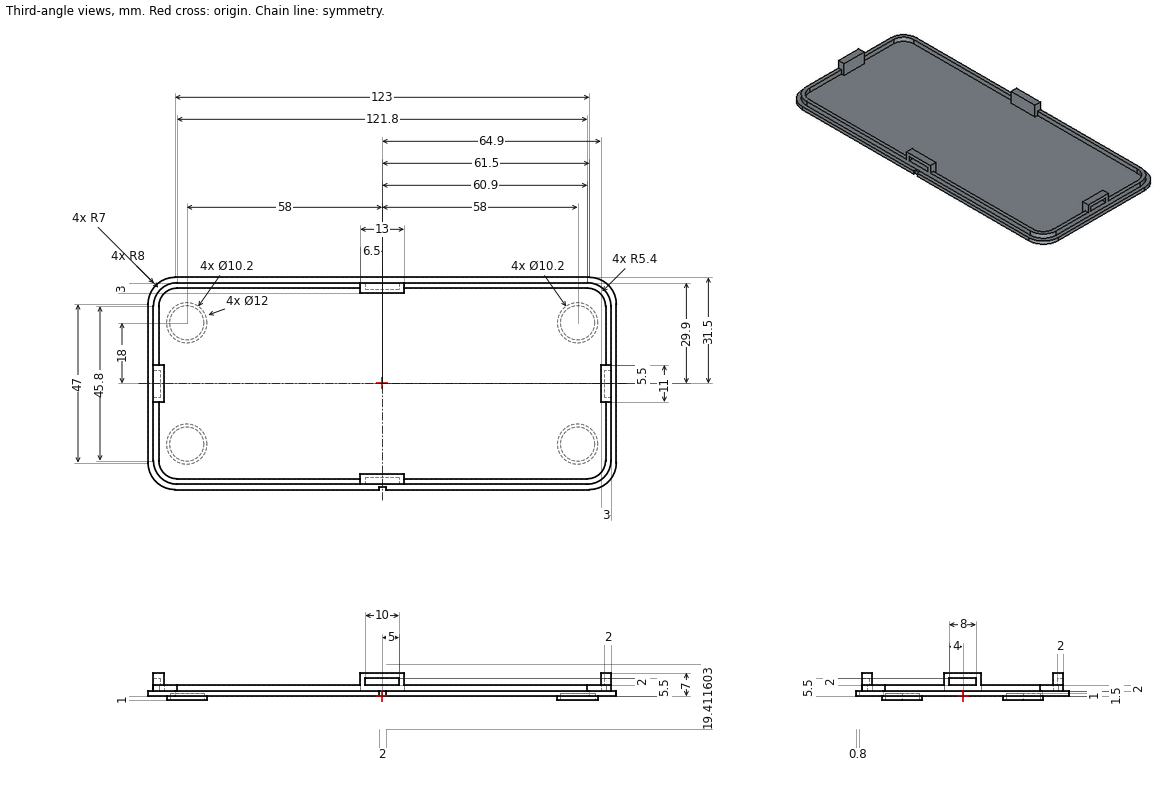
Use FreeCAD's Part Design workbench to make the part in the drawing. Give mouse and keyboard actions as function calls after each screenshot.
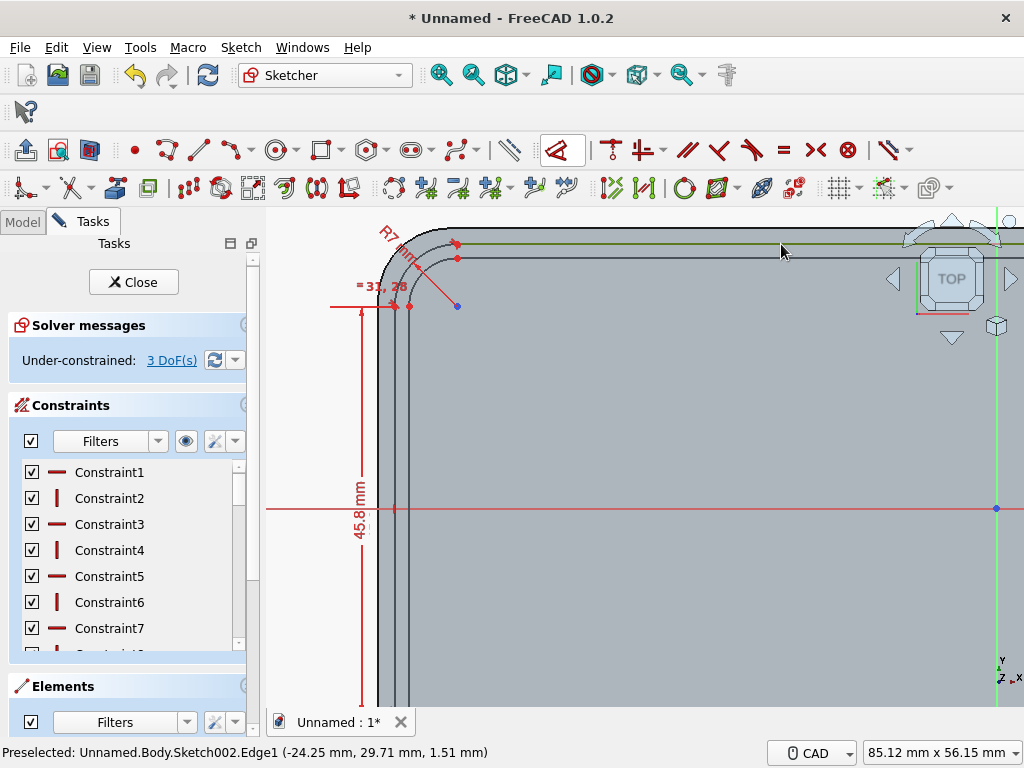
key(l)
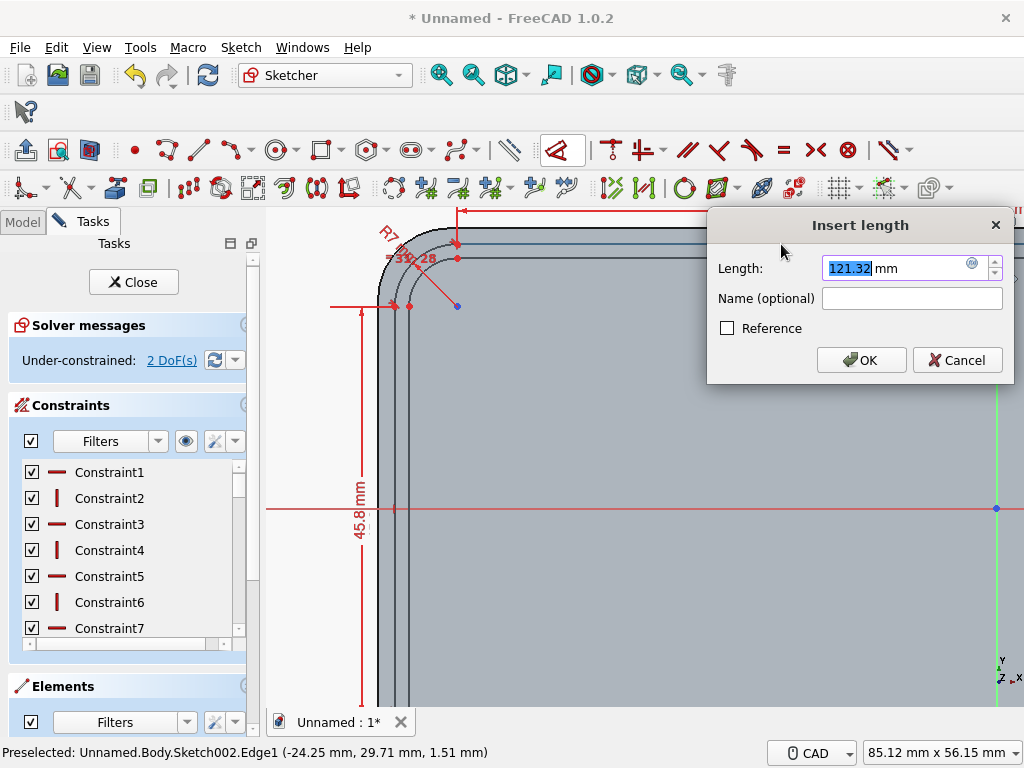
text(121.8)
key(Return)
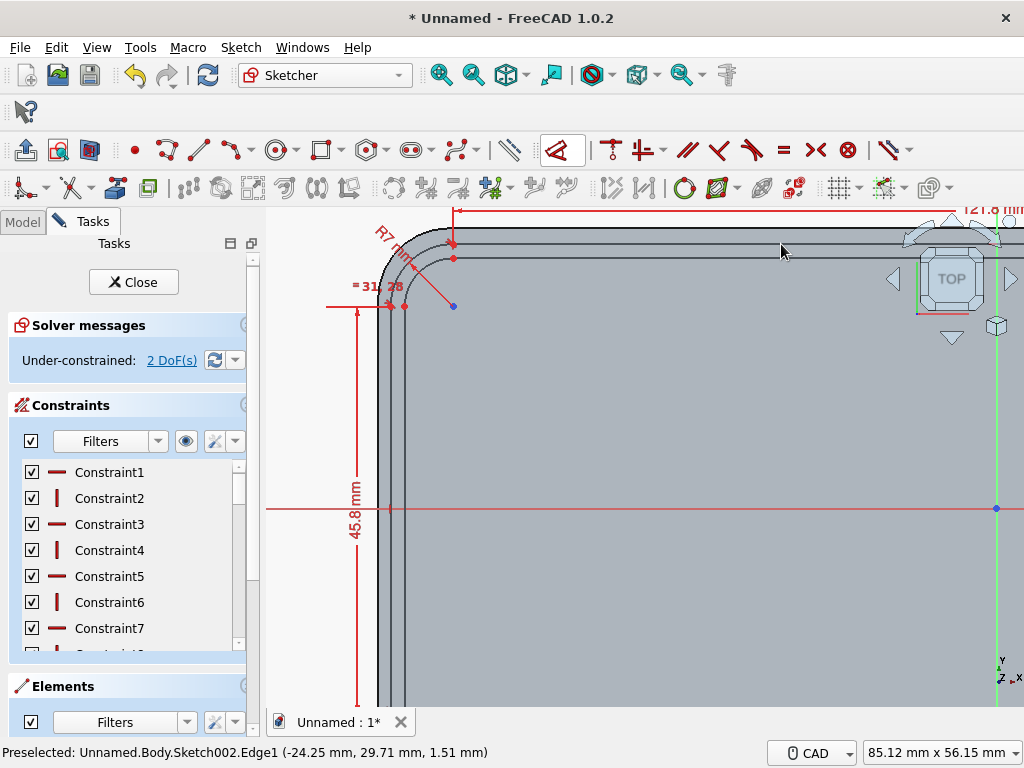
scroll(395, 435, down, 6)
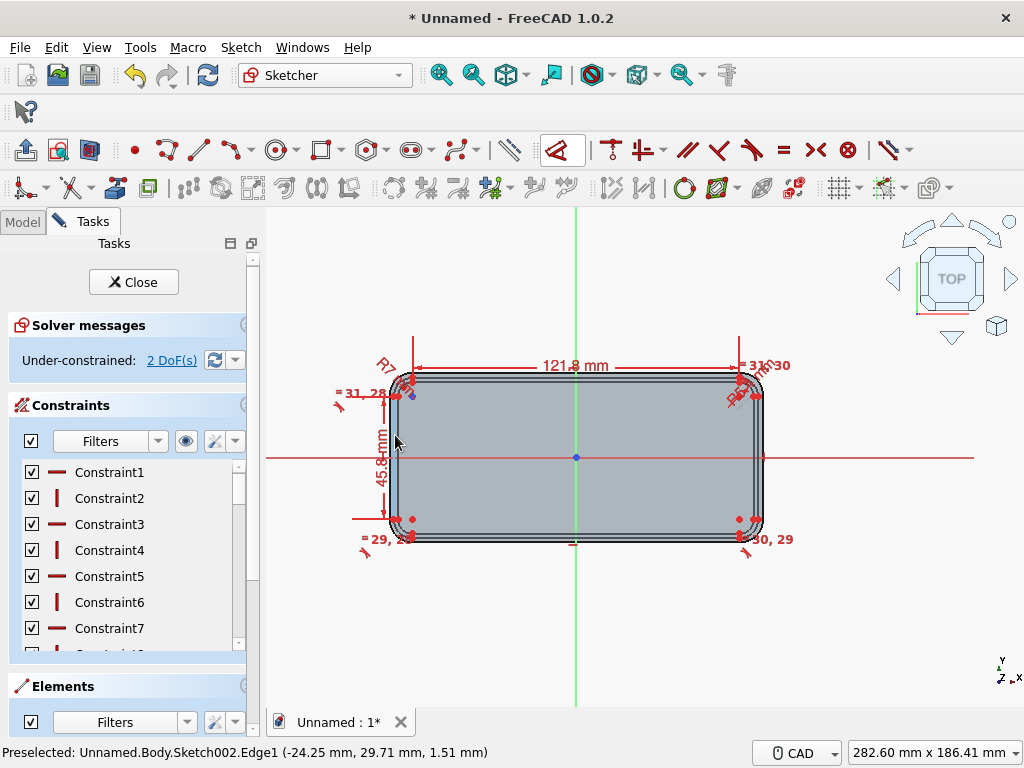
scroll(739, 378, up, 6)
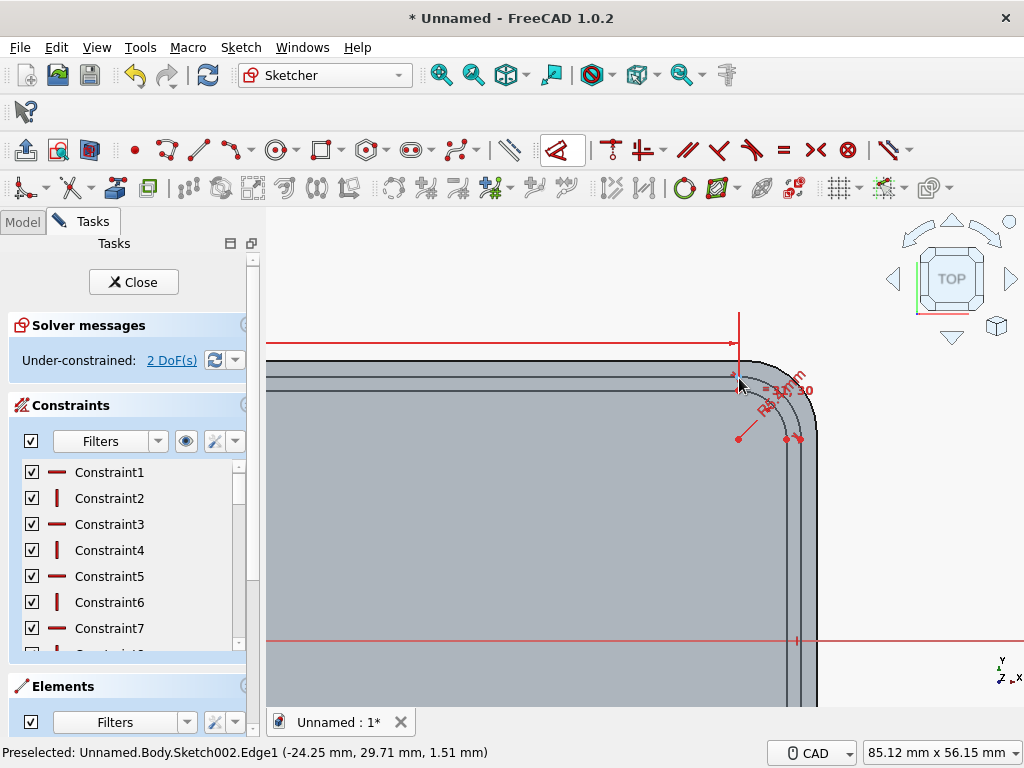
click(739, 377)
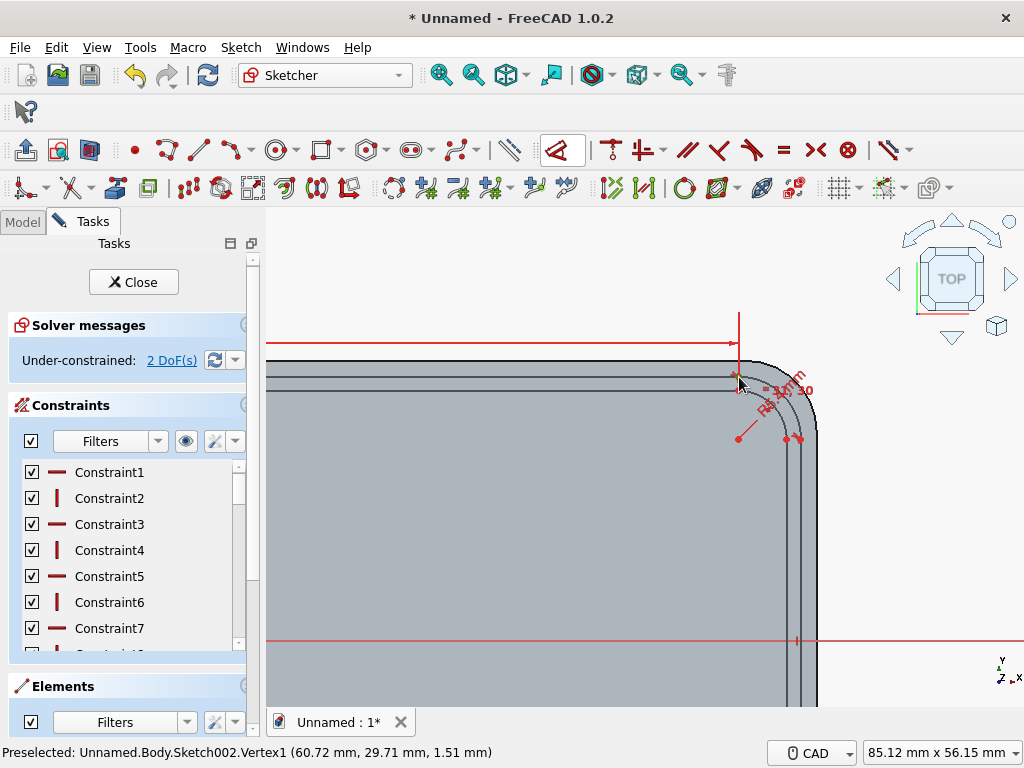
key(l)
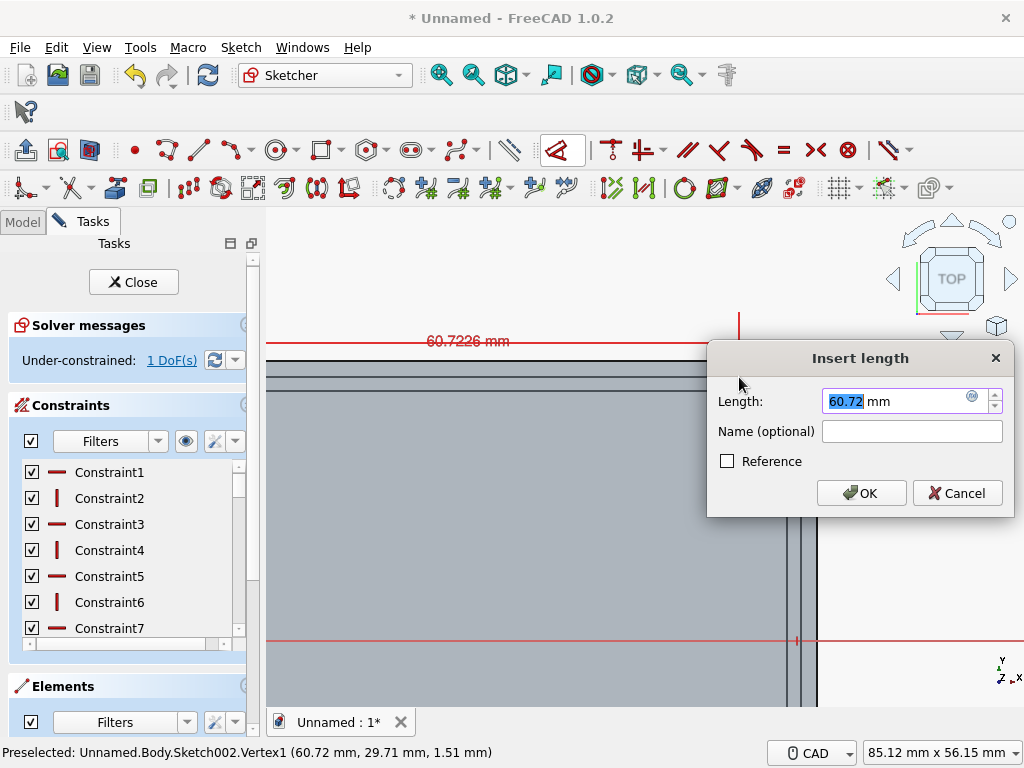
text(60.9)
key(Return)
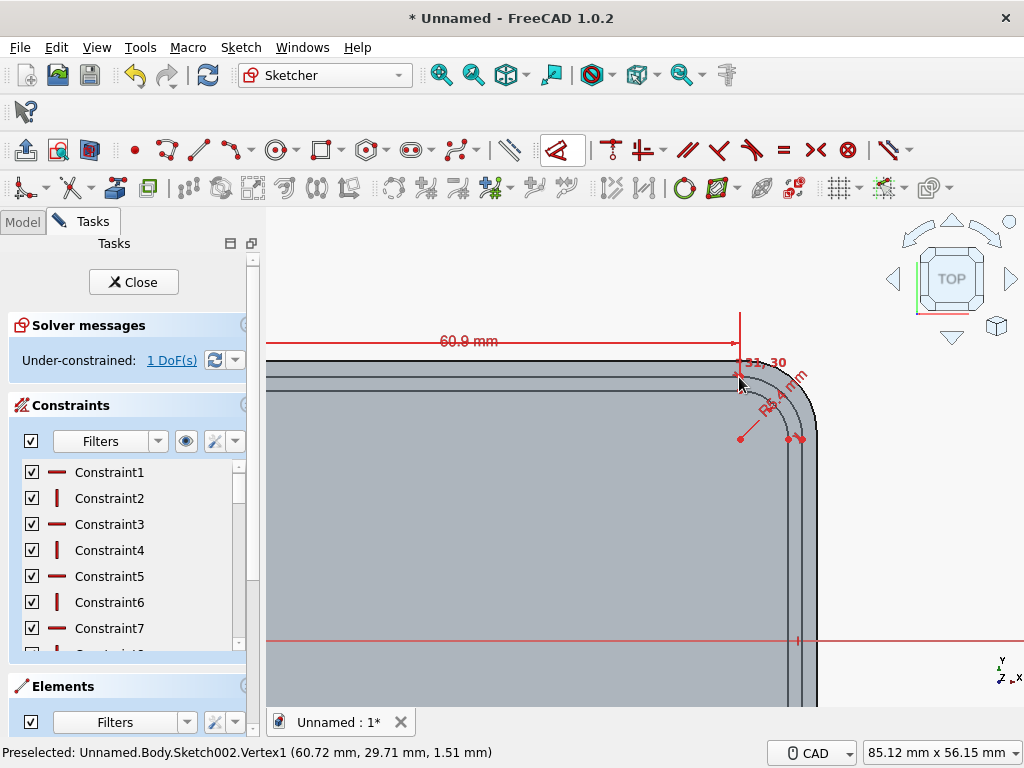
click(740, 377)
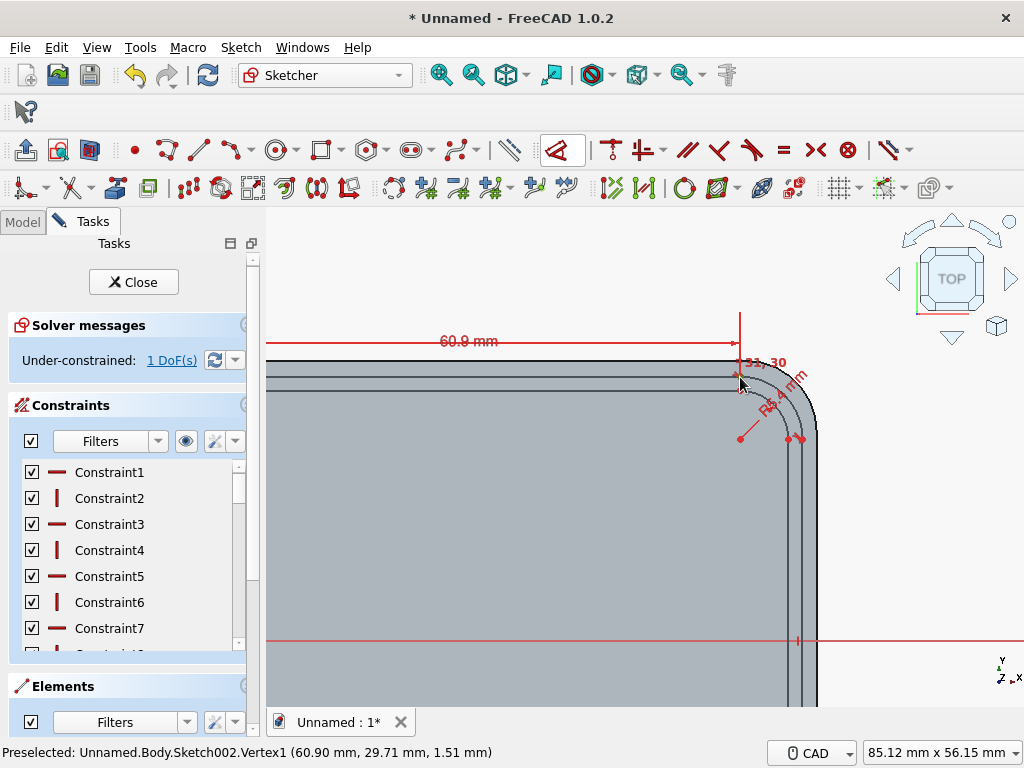
key(i)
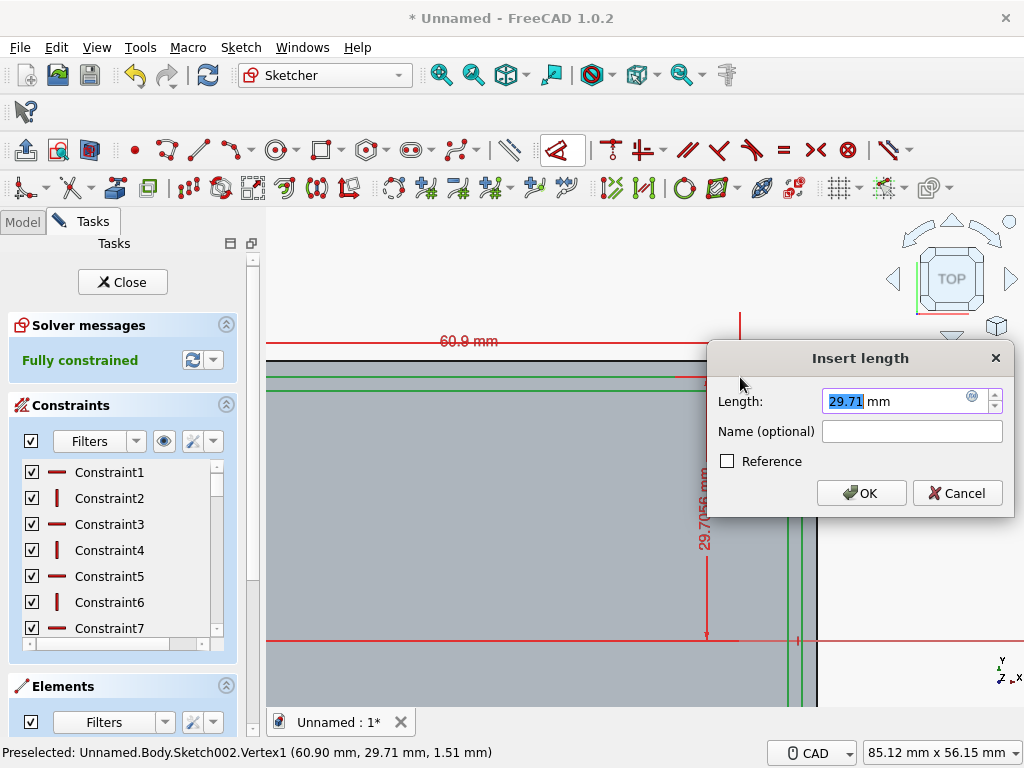
text(29.9)
key(Return)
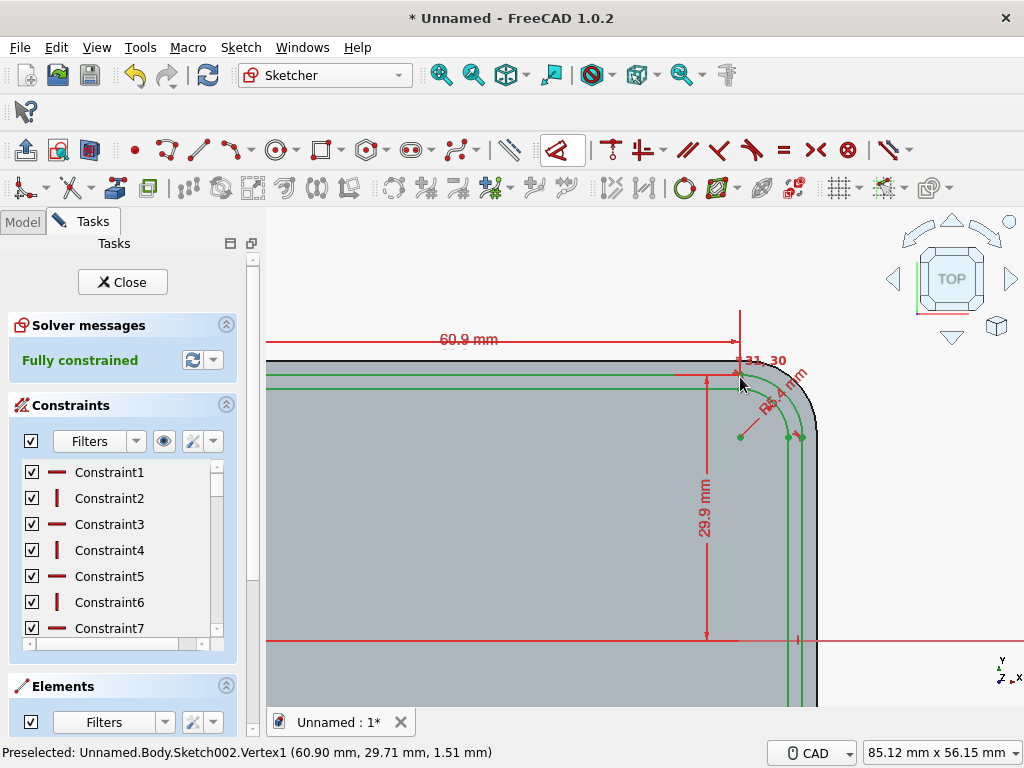
click(123, 282)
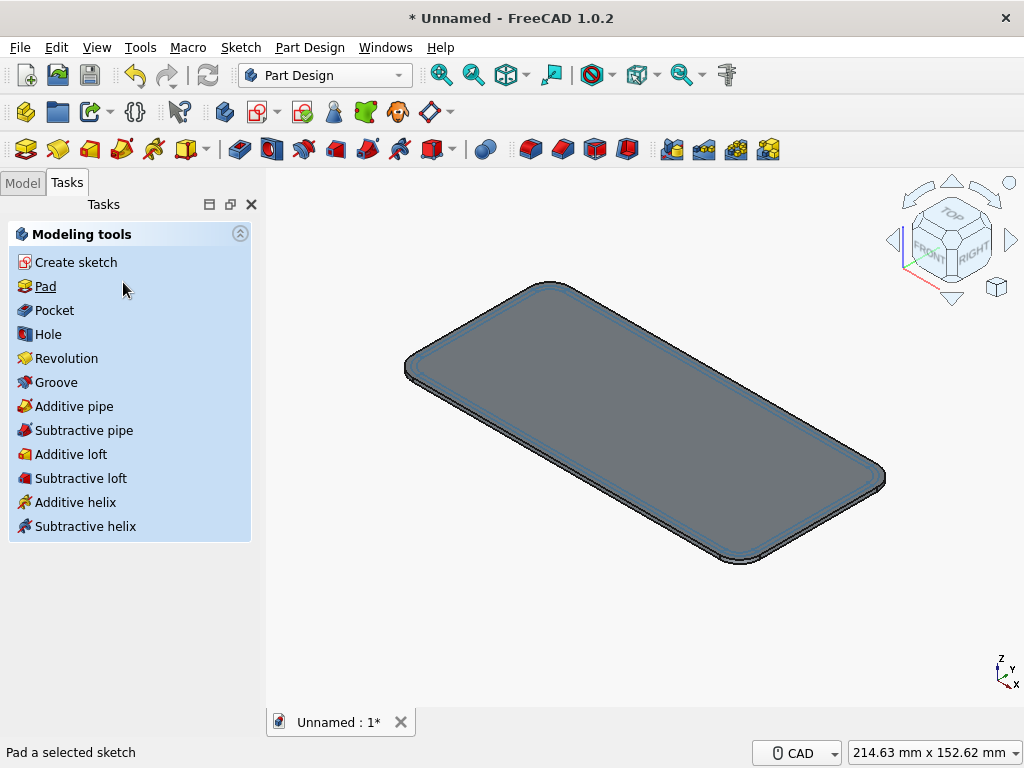
click(26, 150)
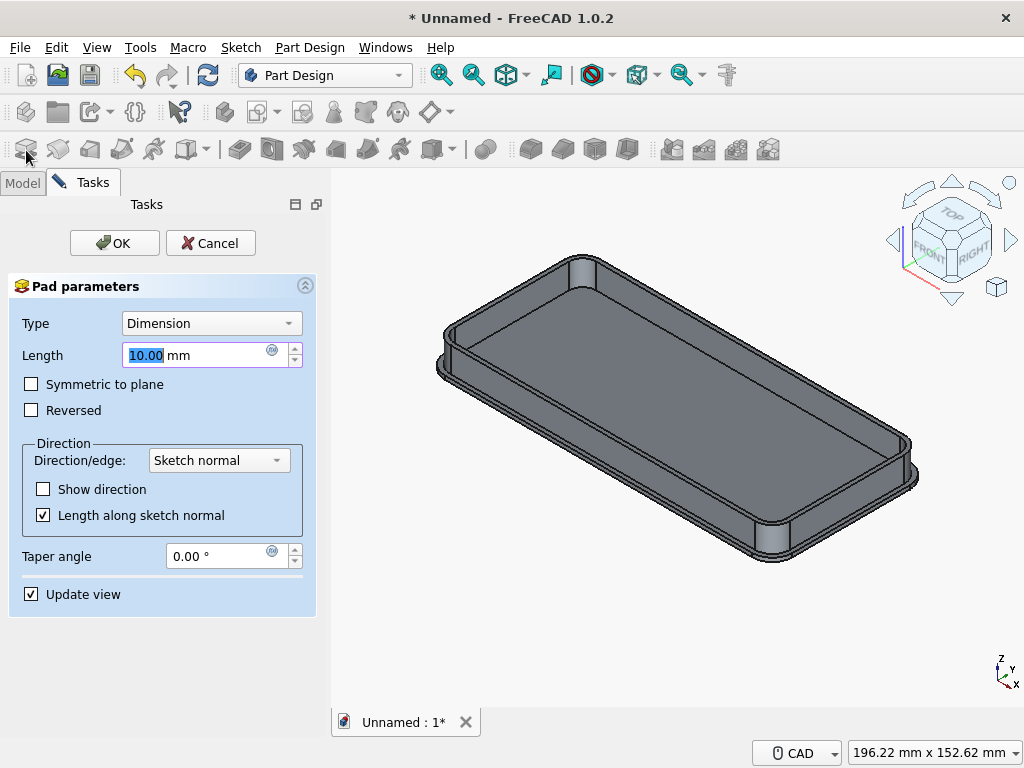
text(2)
key(Tab)